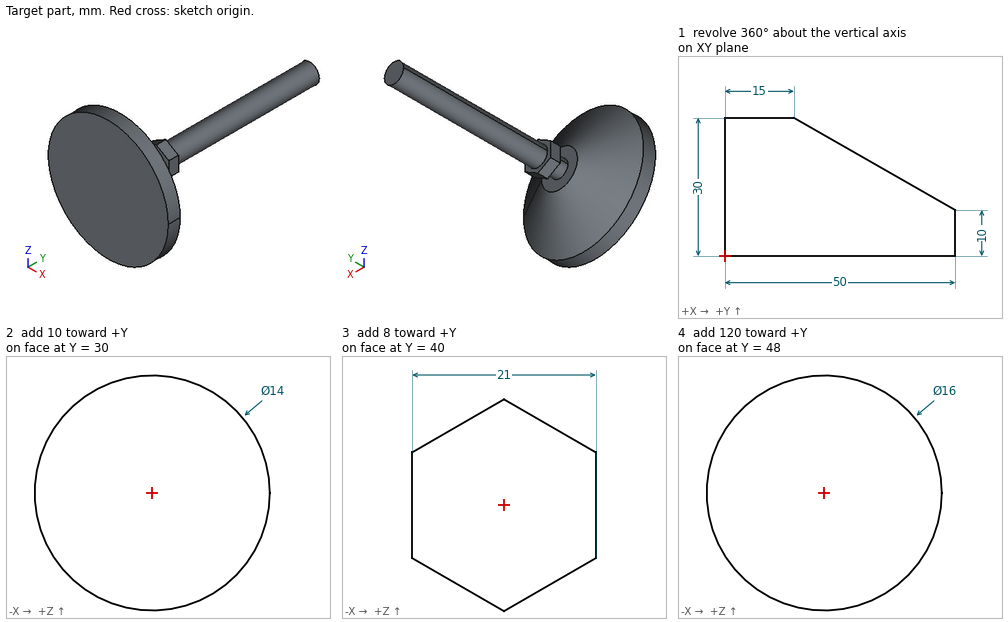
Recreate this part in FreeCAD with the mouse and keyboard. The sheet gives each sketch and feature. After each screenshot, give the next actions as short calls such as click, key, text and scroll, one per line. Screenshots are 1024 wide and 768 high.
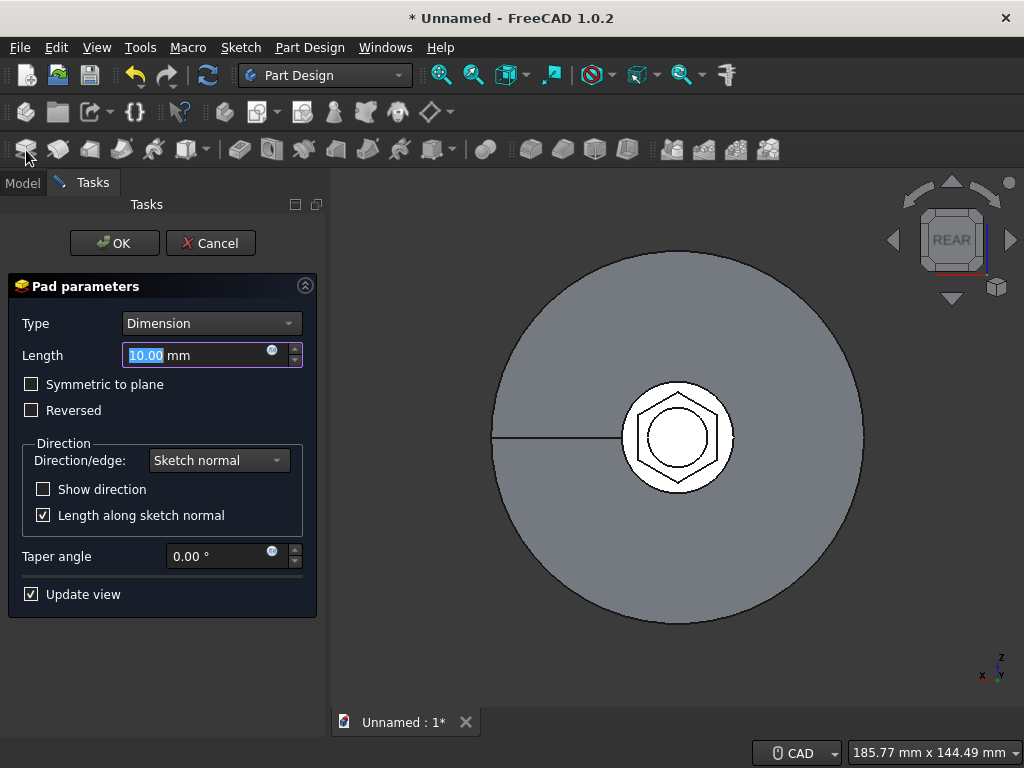
text(120)
key(Tab)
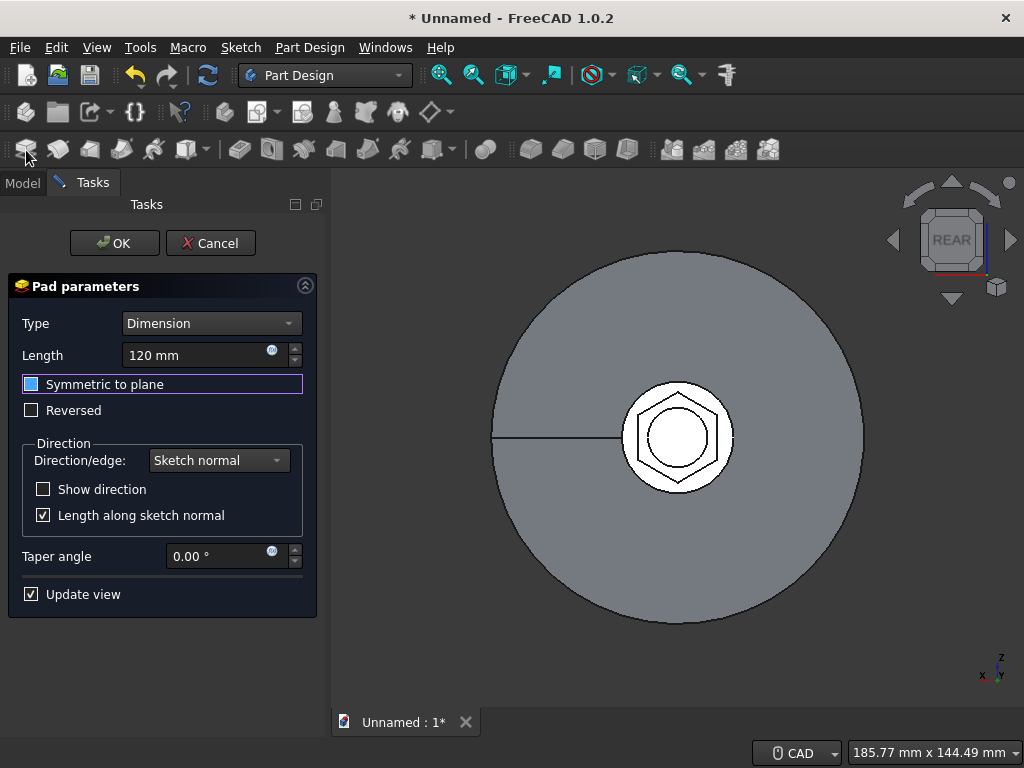
click(115, 243)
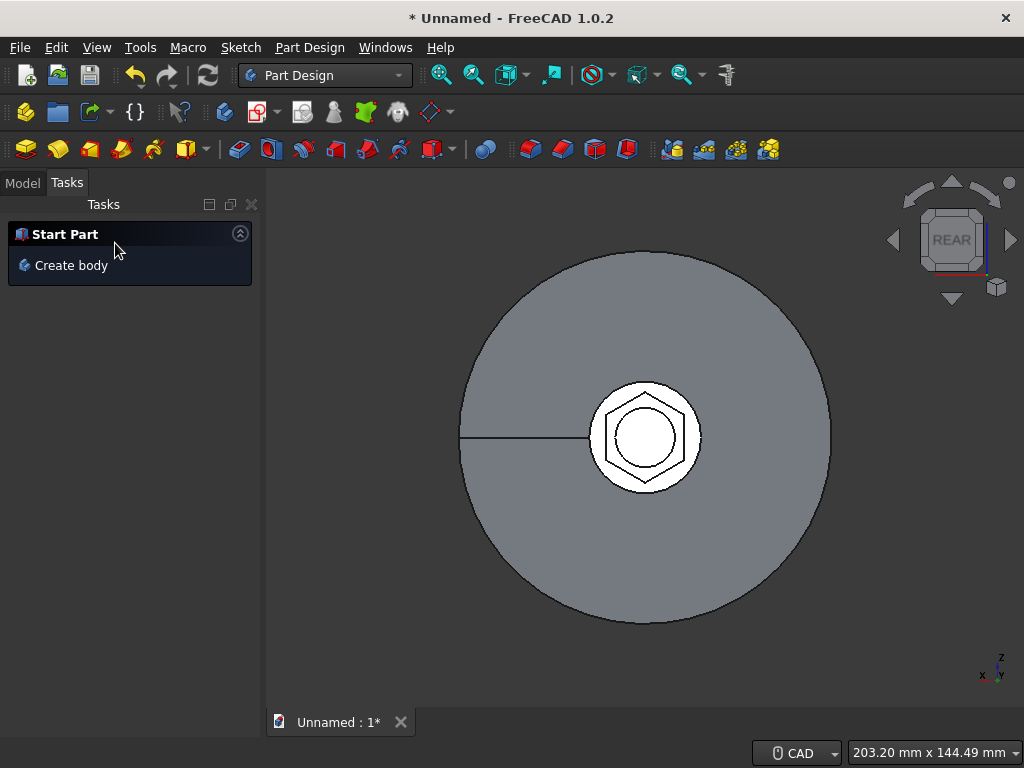
key(0)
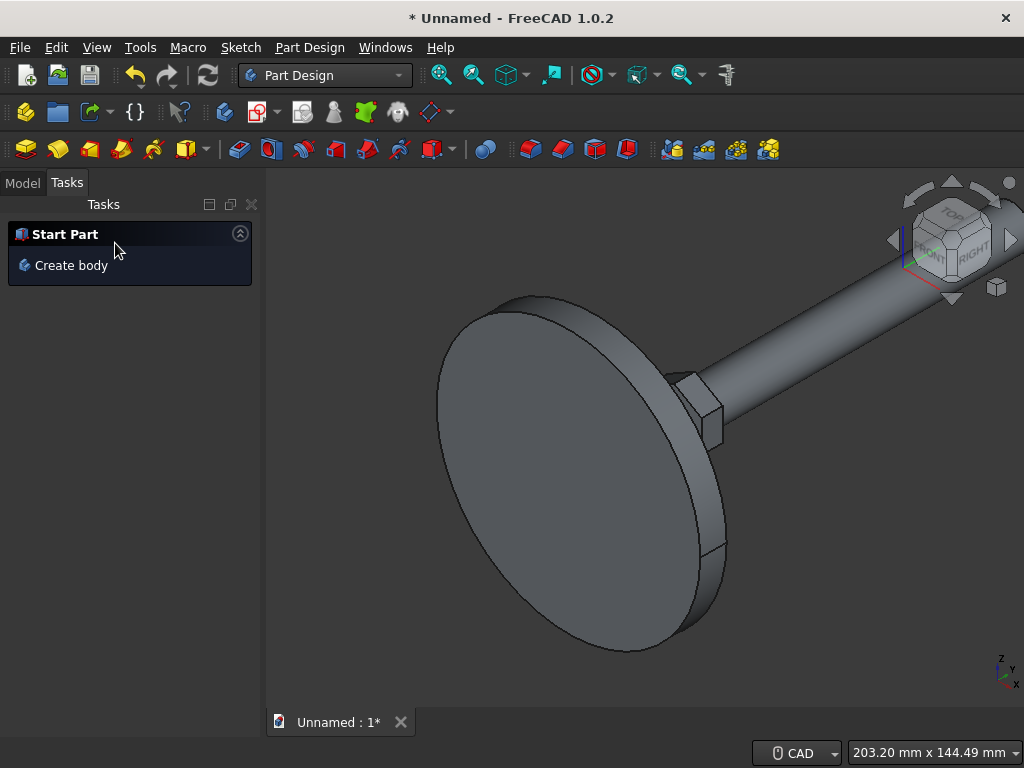
click(442, 76)